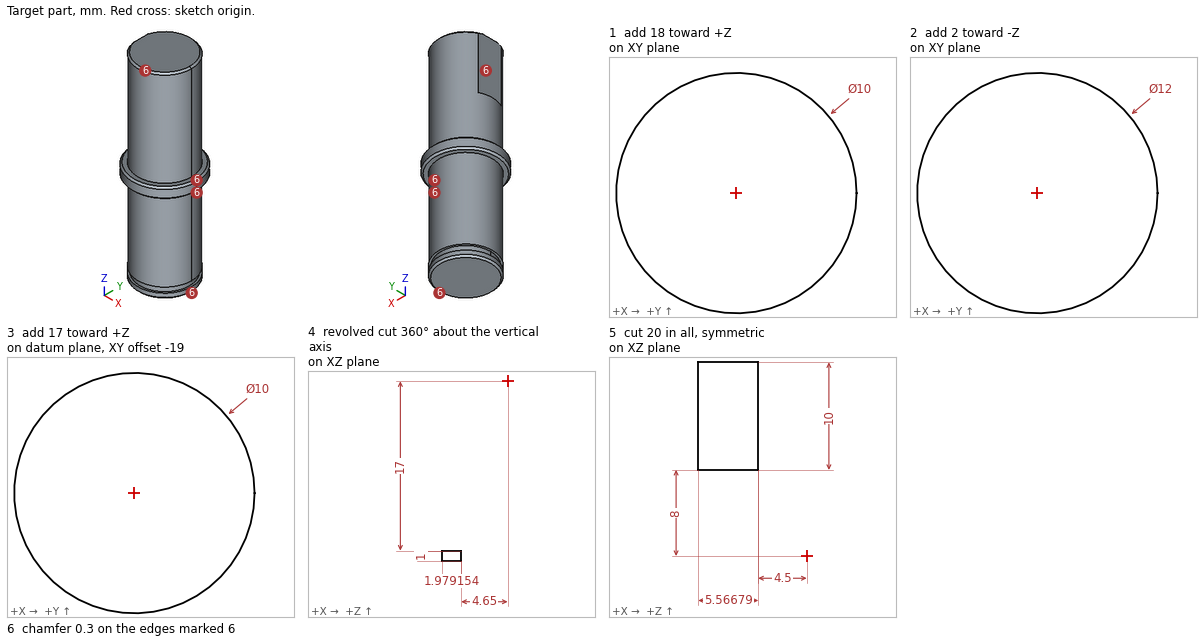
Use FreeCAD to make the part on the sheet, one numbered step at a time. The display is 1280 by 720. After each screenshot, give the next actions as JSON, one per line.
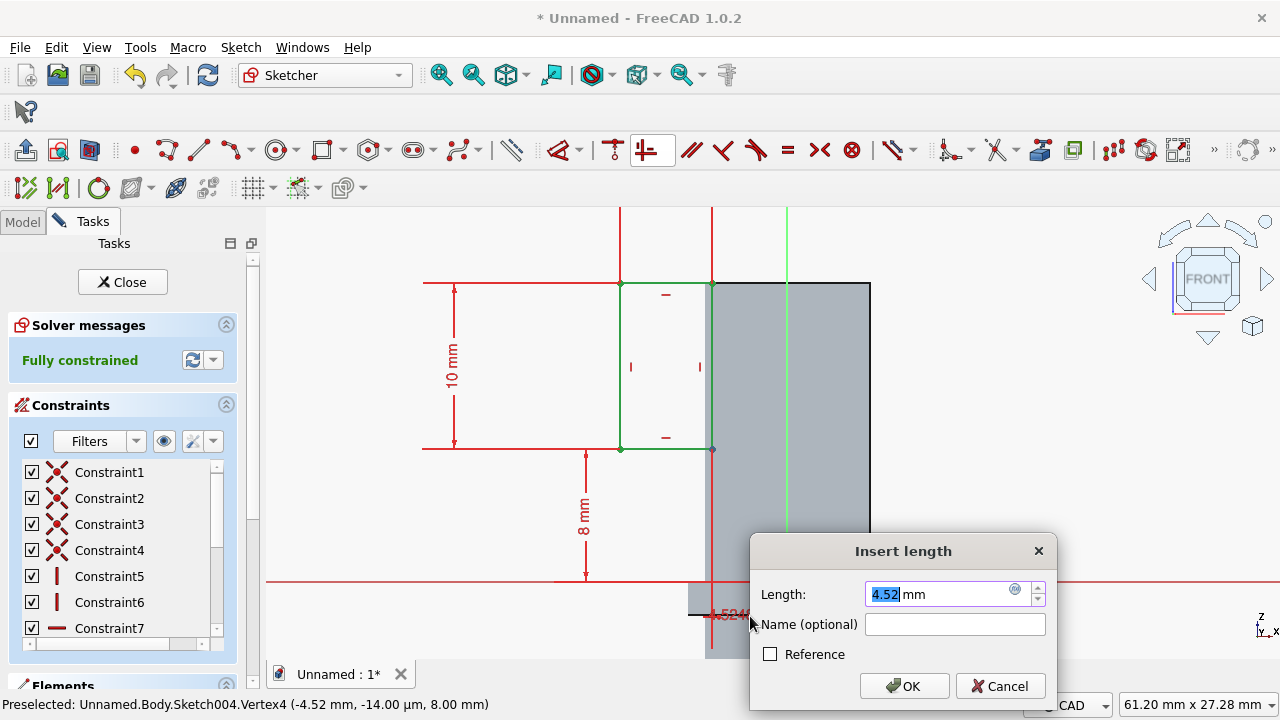
{"action": "type", "text": "4.5"}
{"action": "key", "text": "Return"}
{"action": "key", "text": "Escape"}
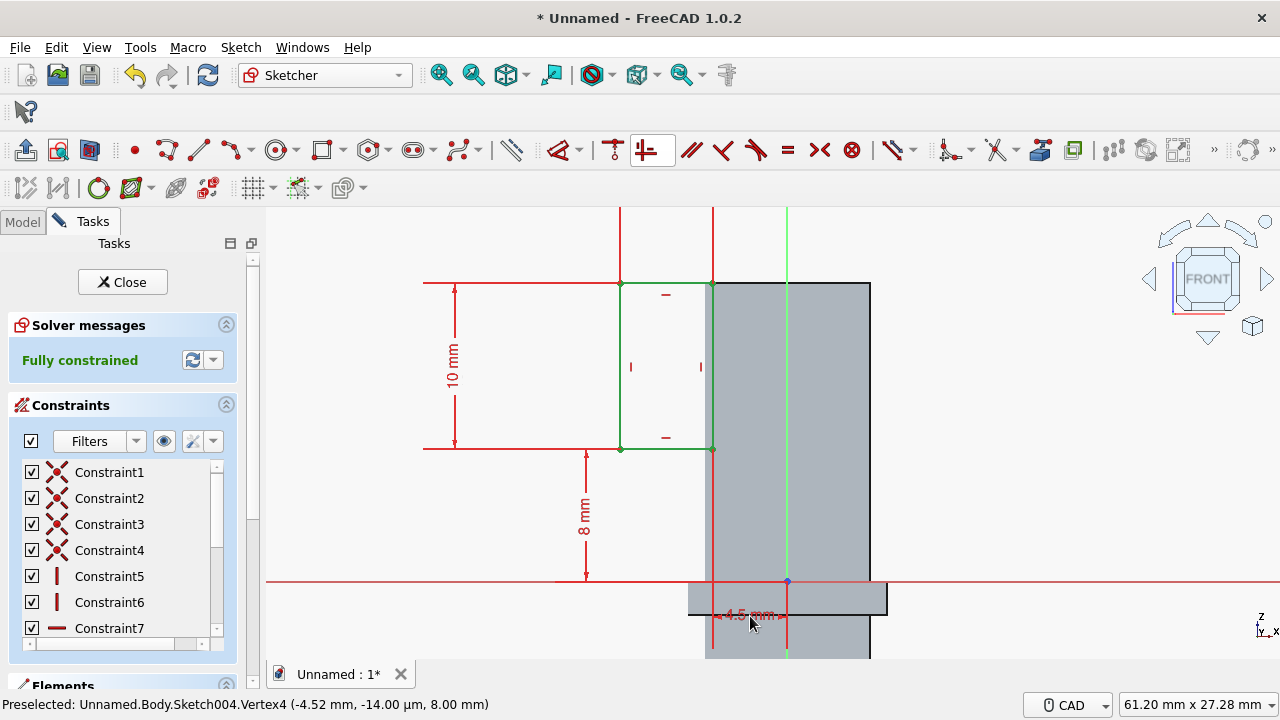
{"action": "left_click", "coordinate": [123, 282]}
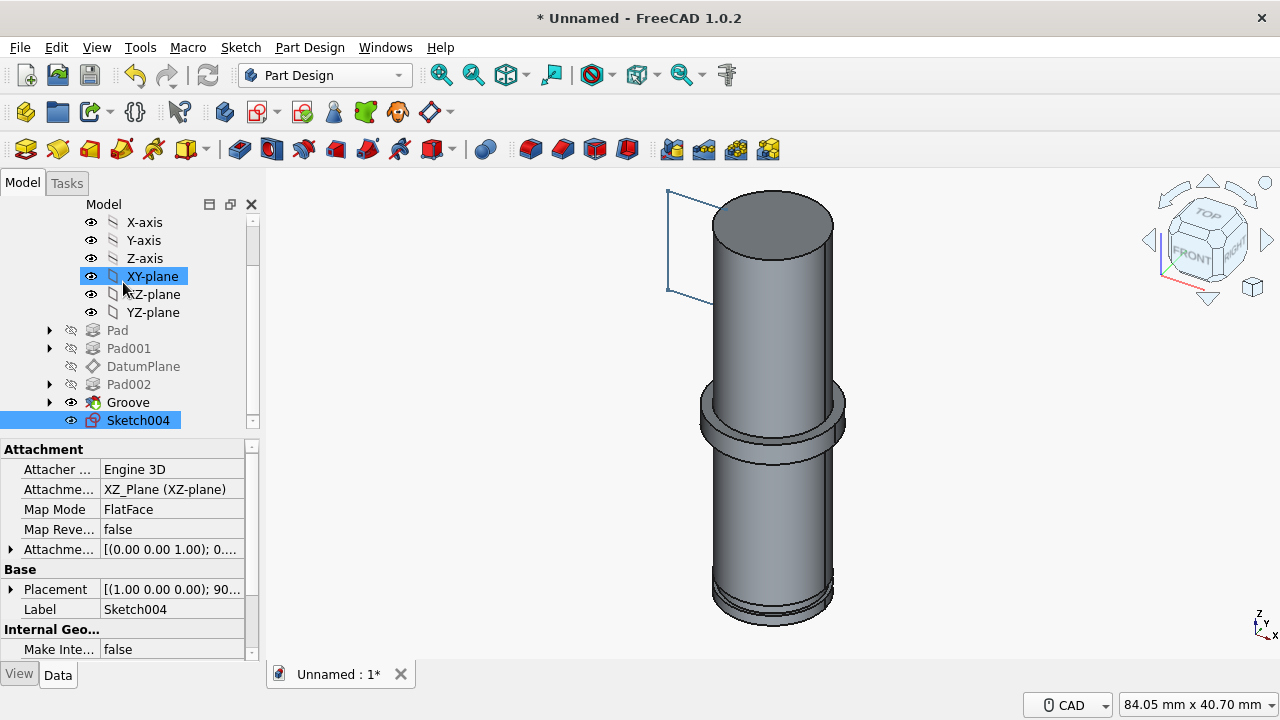
{"action": "left_click", "coordinate": [240, 150]}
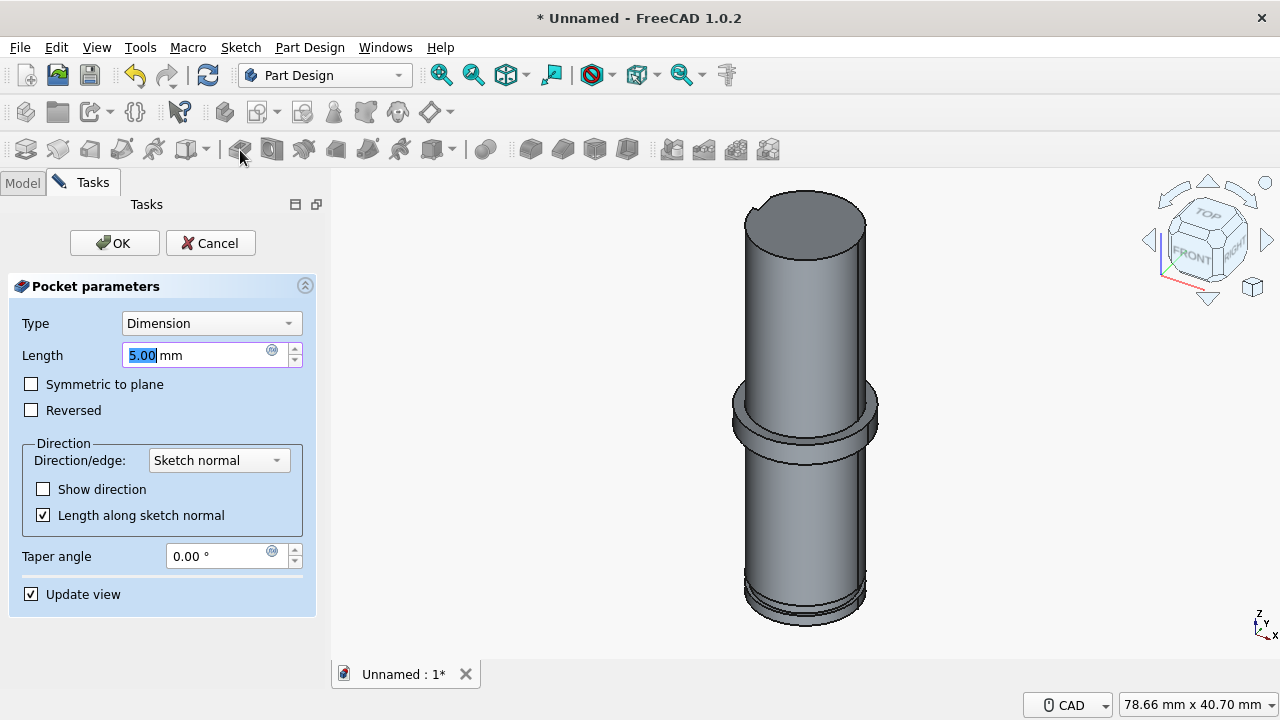
{"action": "type", "text": "20"}
{"action": "key", "text": "Tab"}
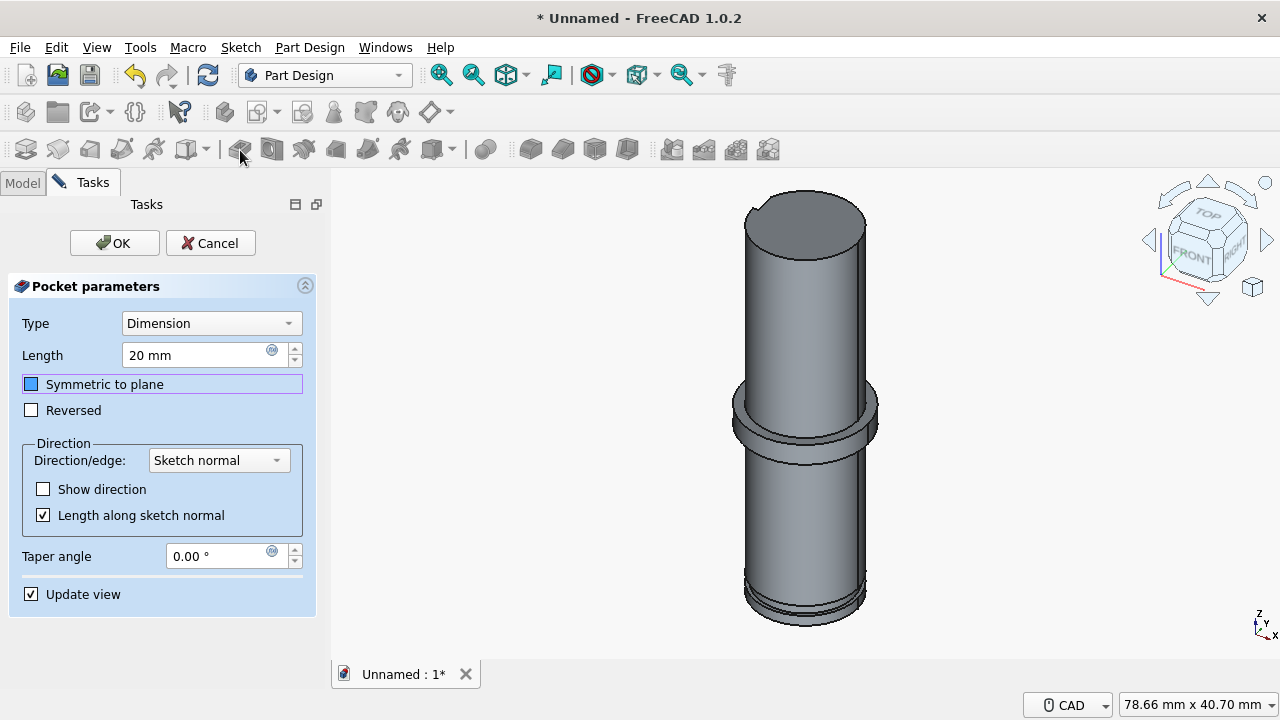
{"action": "left_click", "coordinate": [30, 384]}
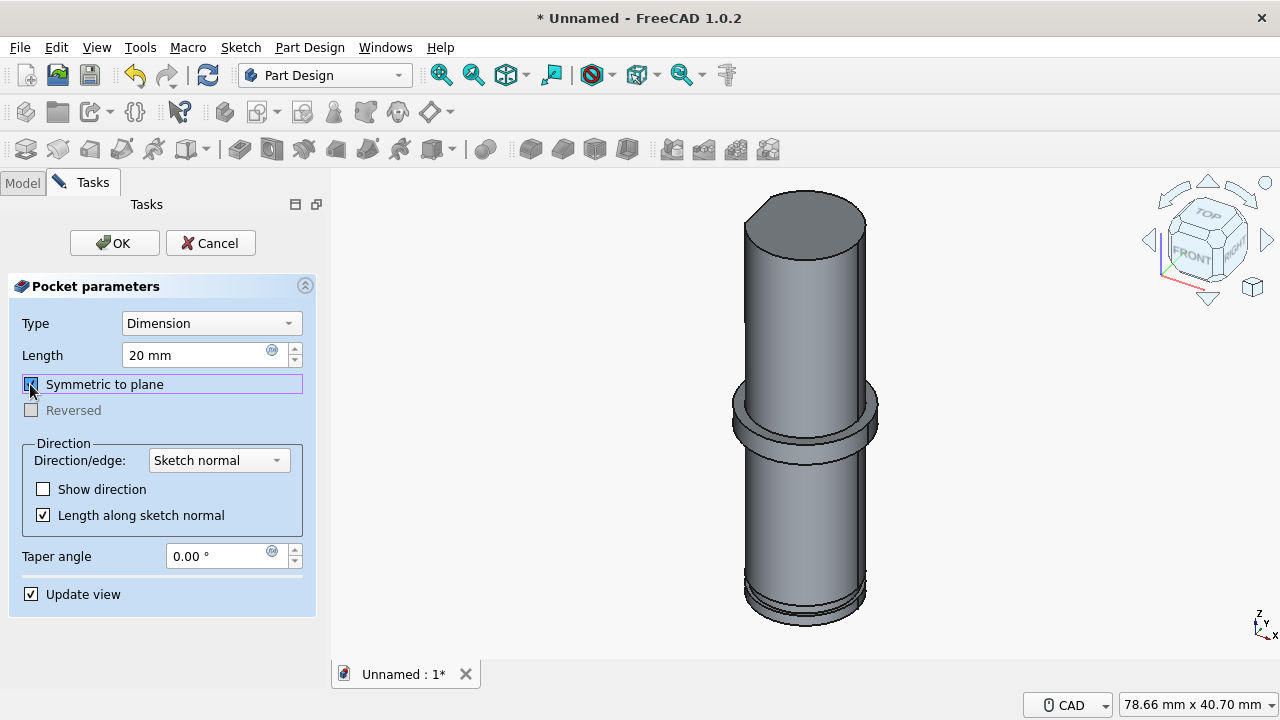
{"action": "left_click", "coordinate": [115, 243]}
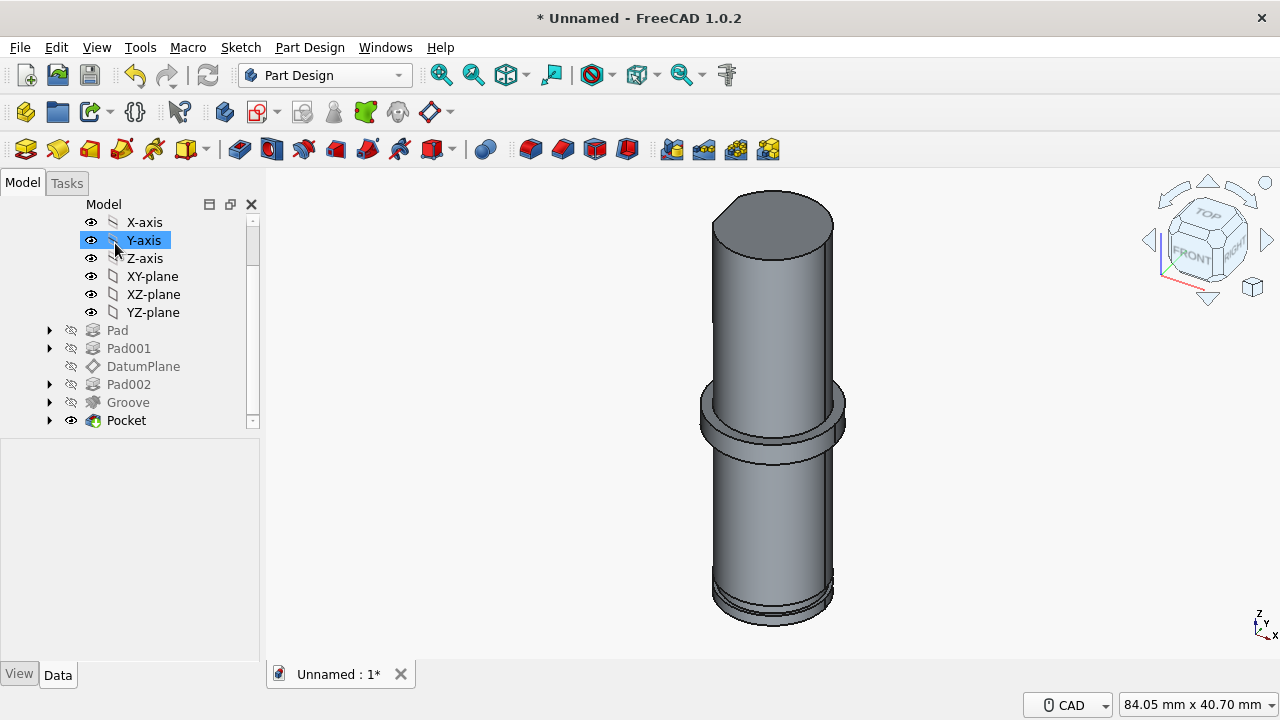
{"action": "left_click", "coordinate": [755, 258]}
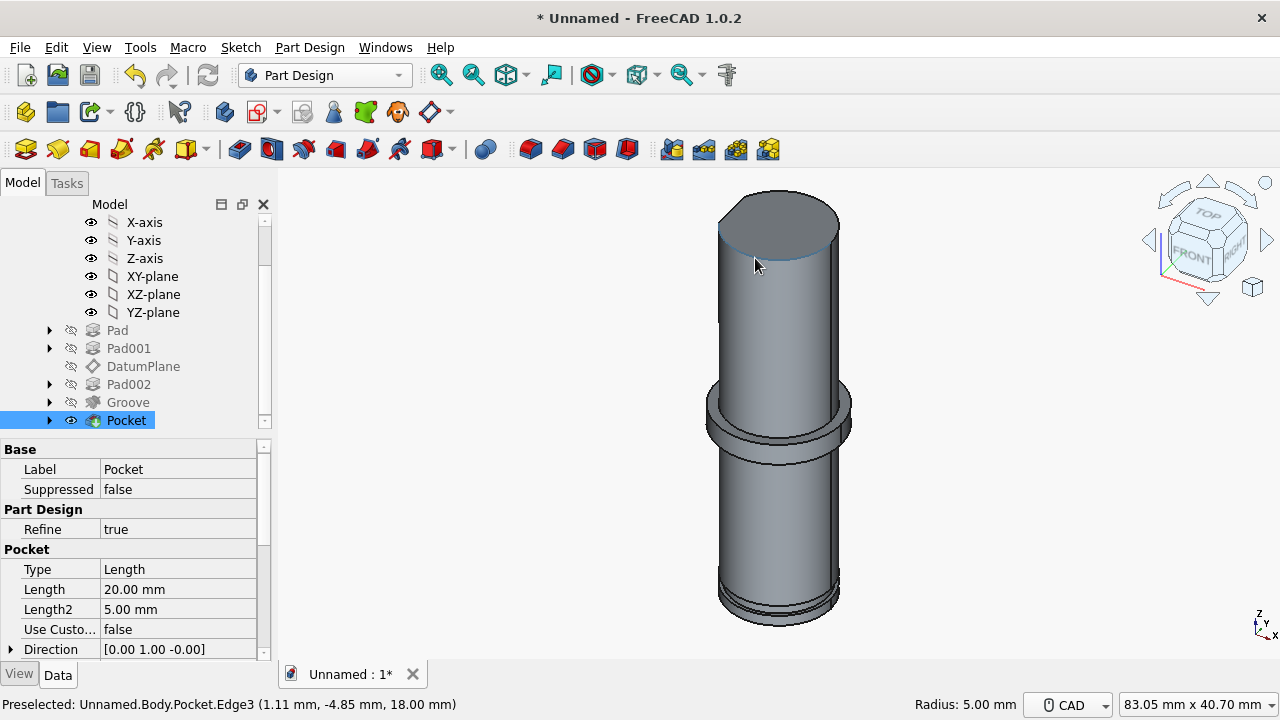
{"action": "left_click", "coordinate": [707, 407], "text": "ctrl"}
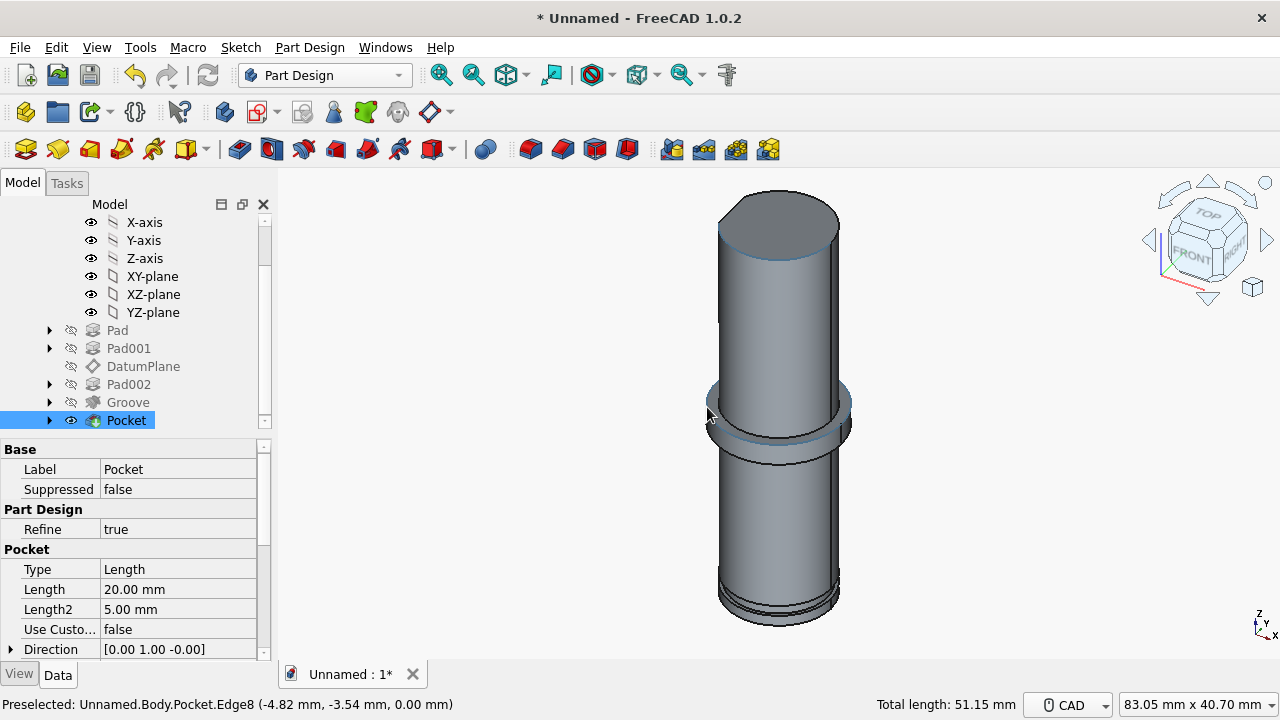
{"action": "key", "text": "0"}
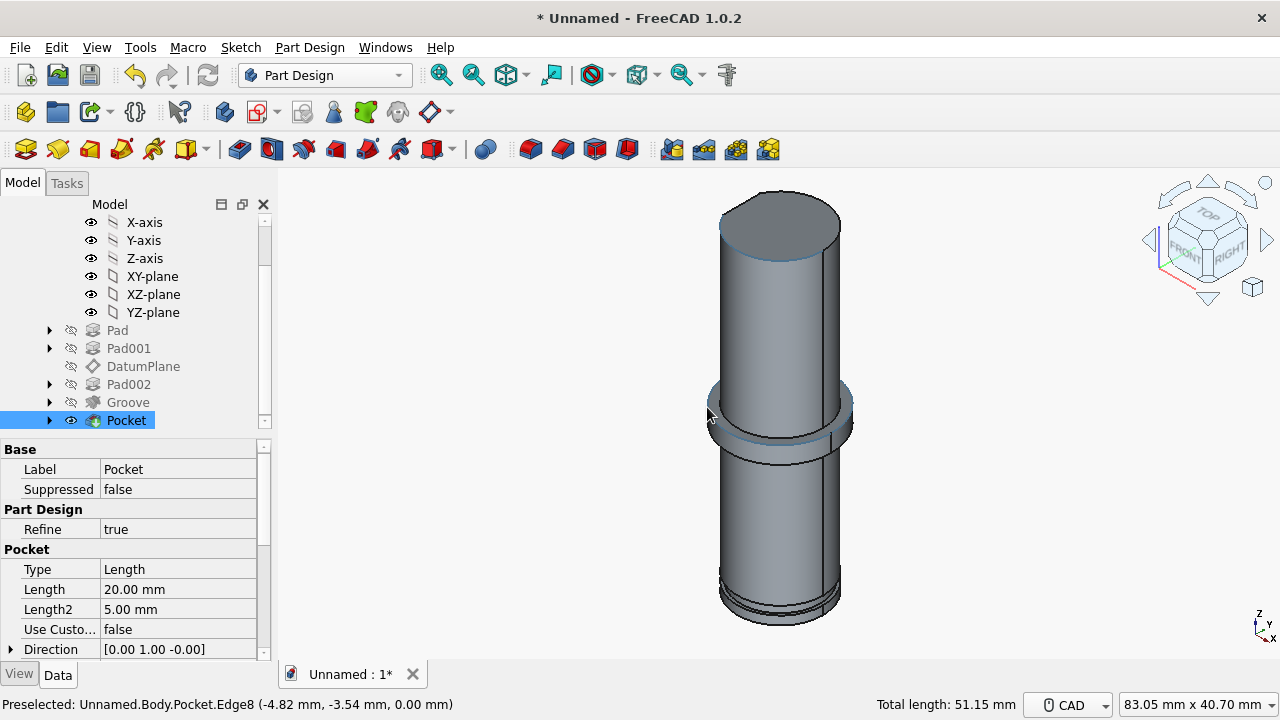
{"action": "left_click", "coordinate": [442, 76]}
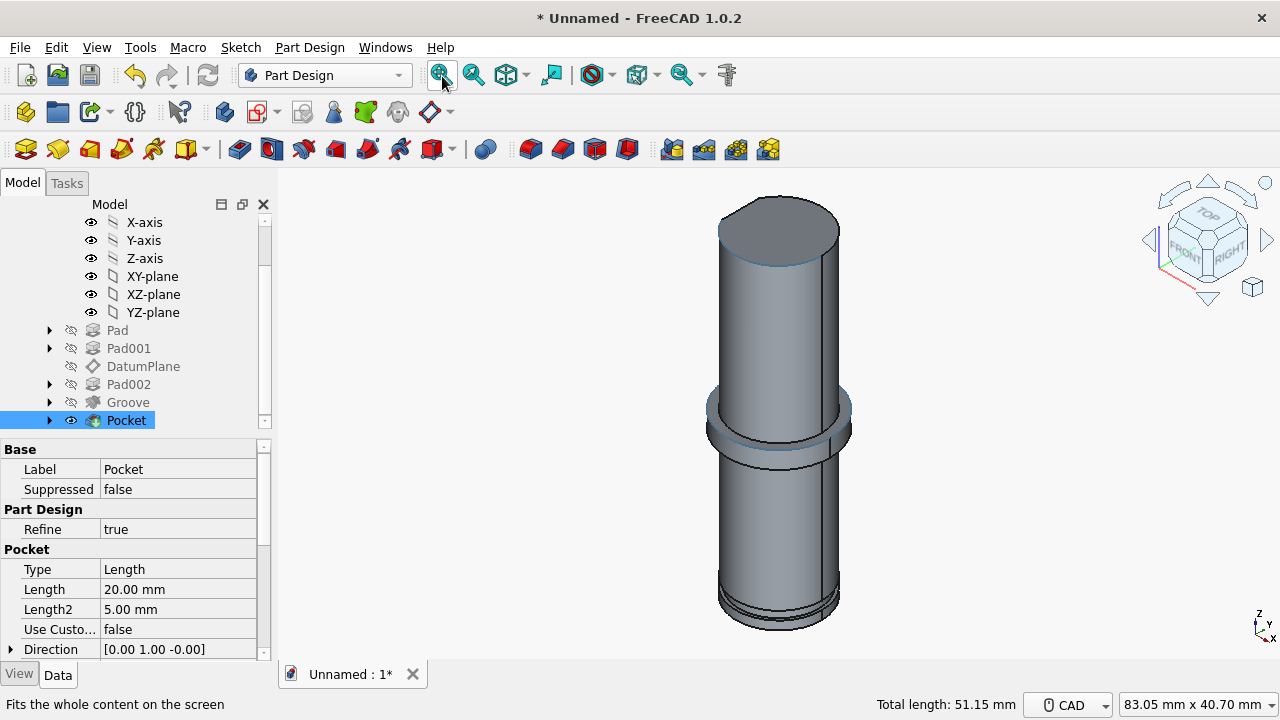
{"action": "left_click", "coordinate": [725, 611], "text": "ctrl"}